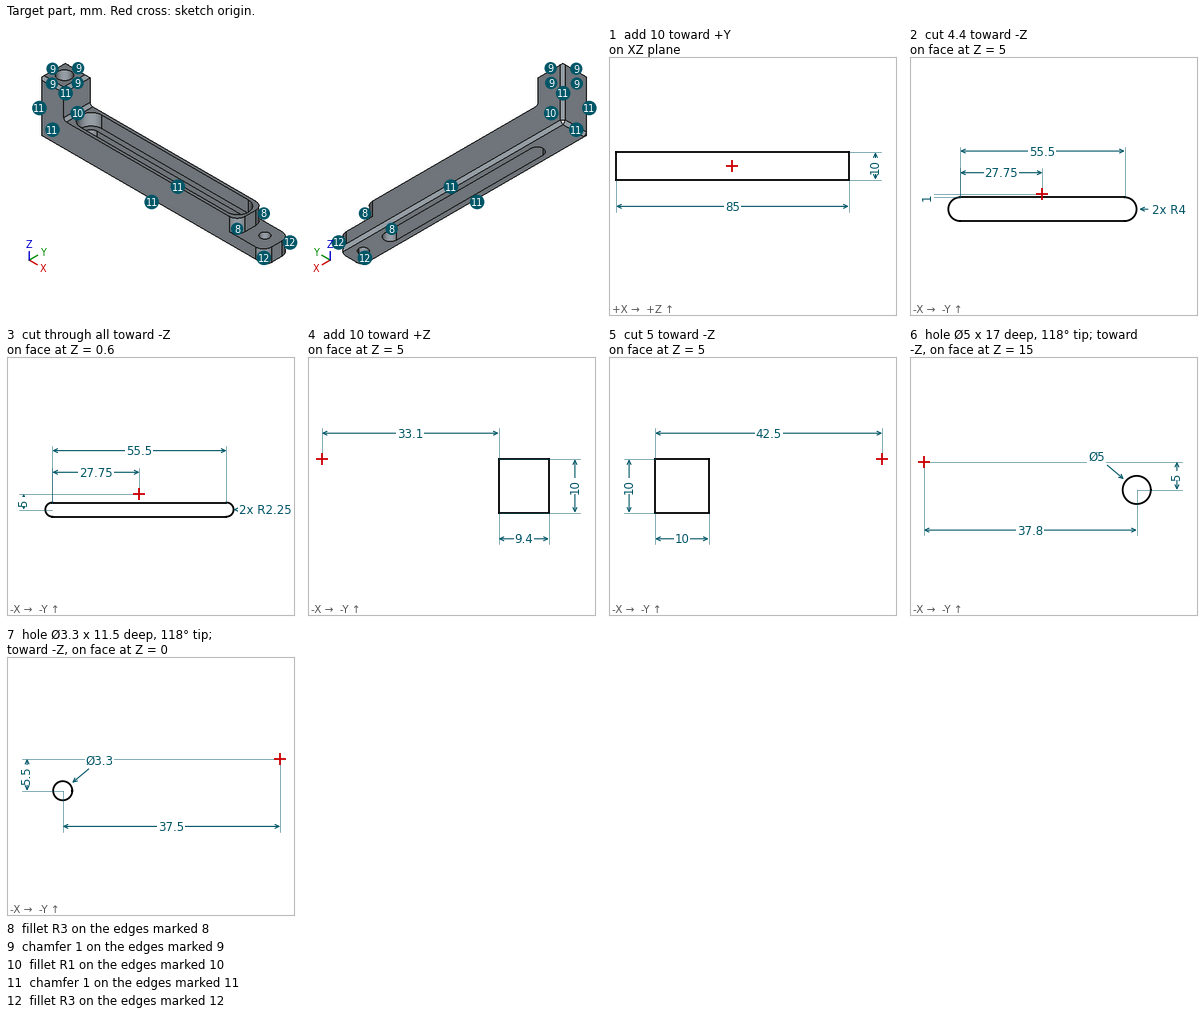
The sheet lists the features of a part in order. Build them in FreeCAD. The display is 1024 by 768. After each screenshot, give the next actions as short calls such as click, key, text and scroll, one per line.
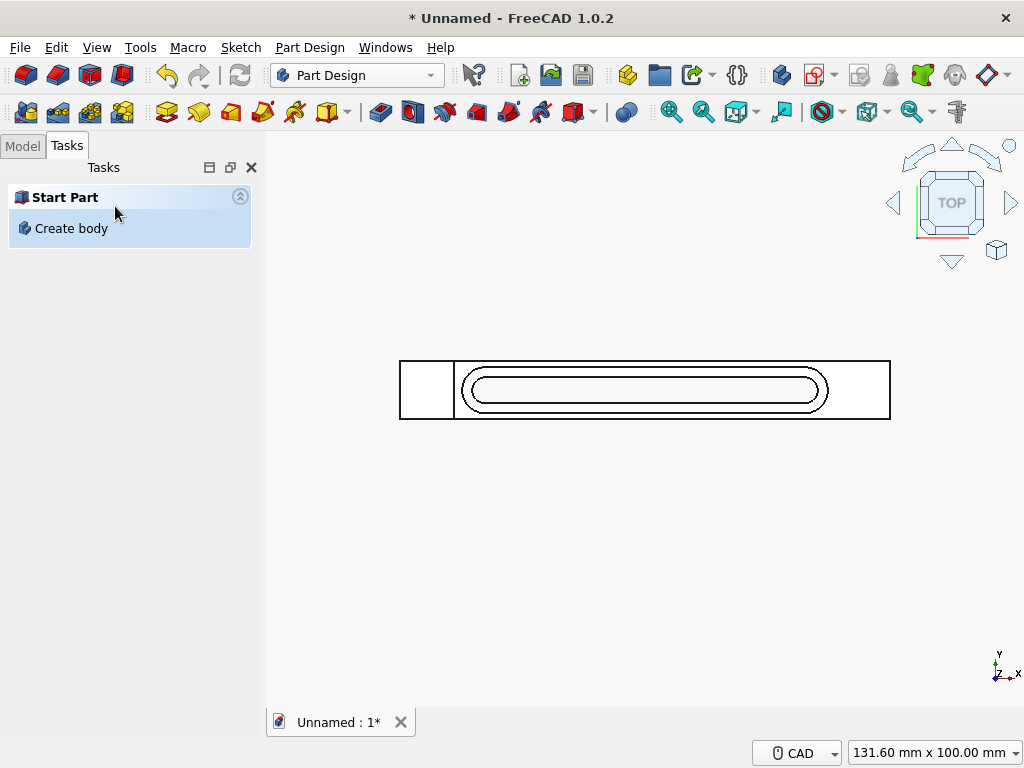
click(859, 389)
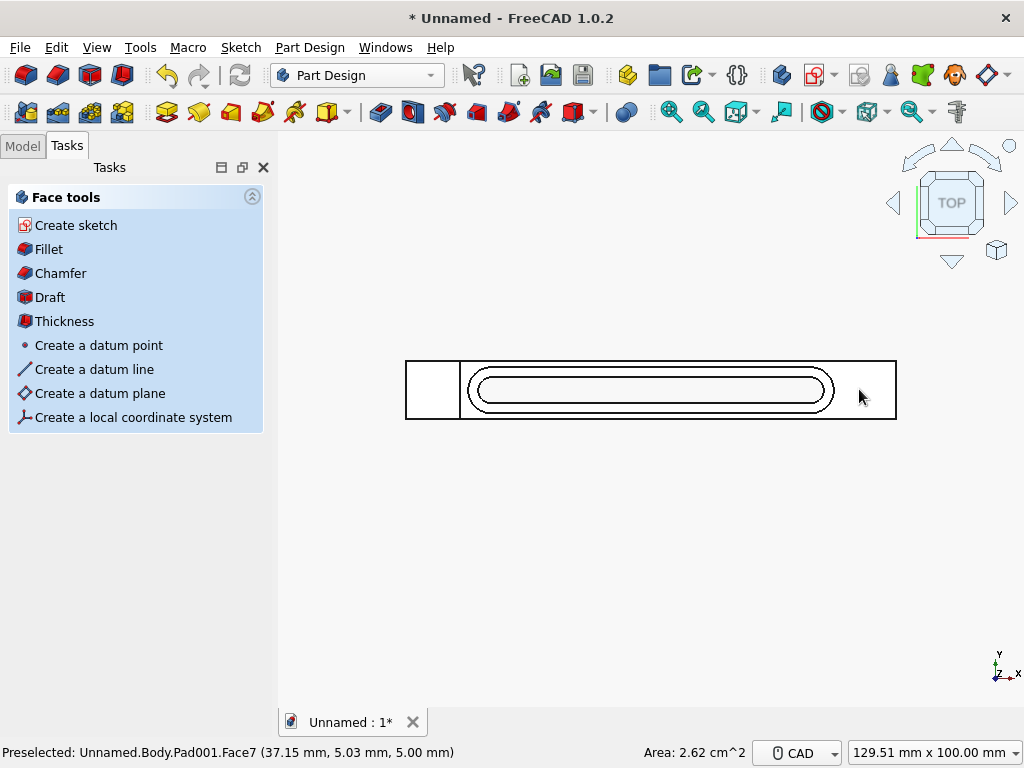
click(814, 76)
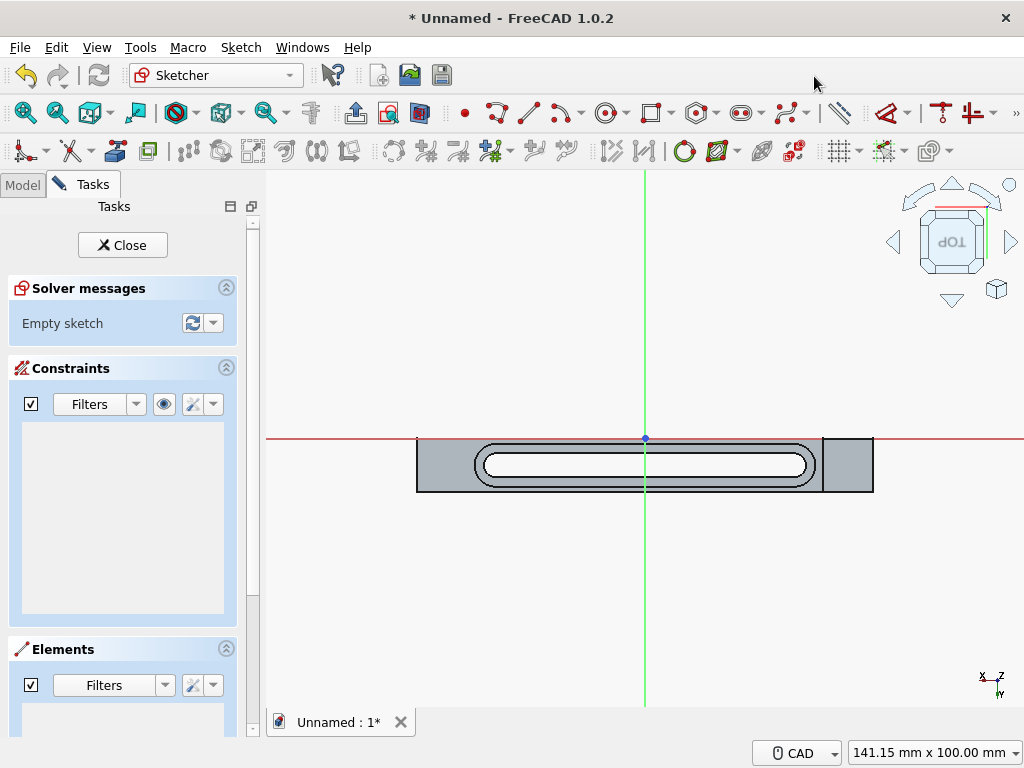
click(420, 114)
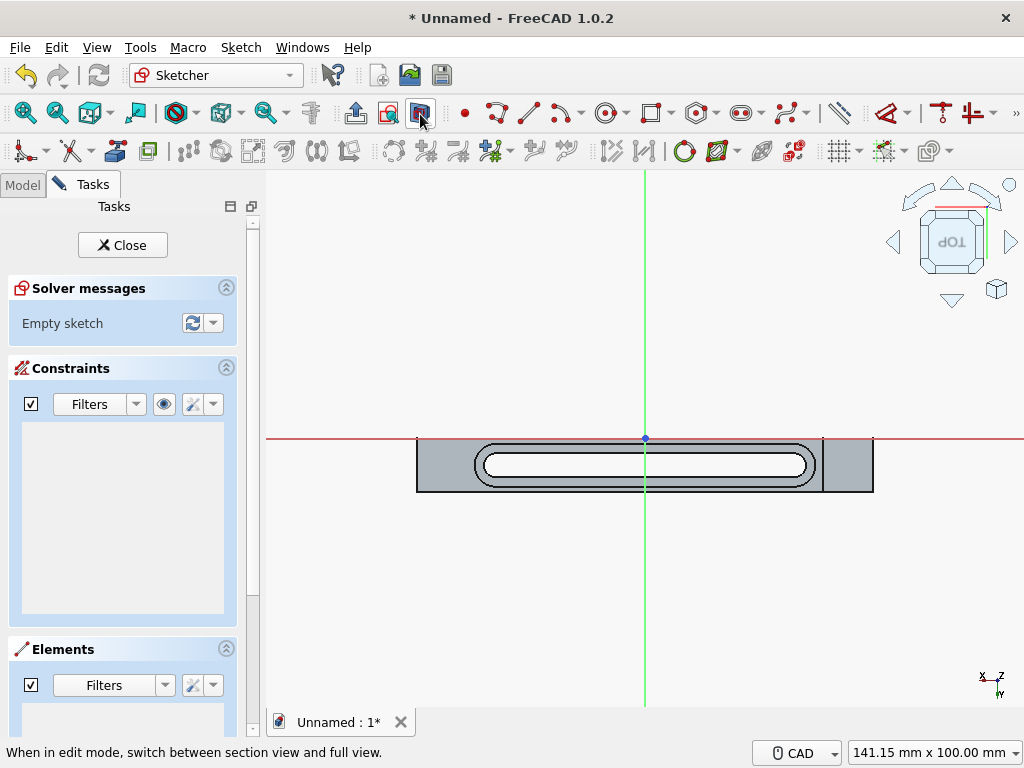
scroll(417, 471, up, 9)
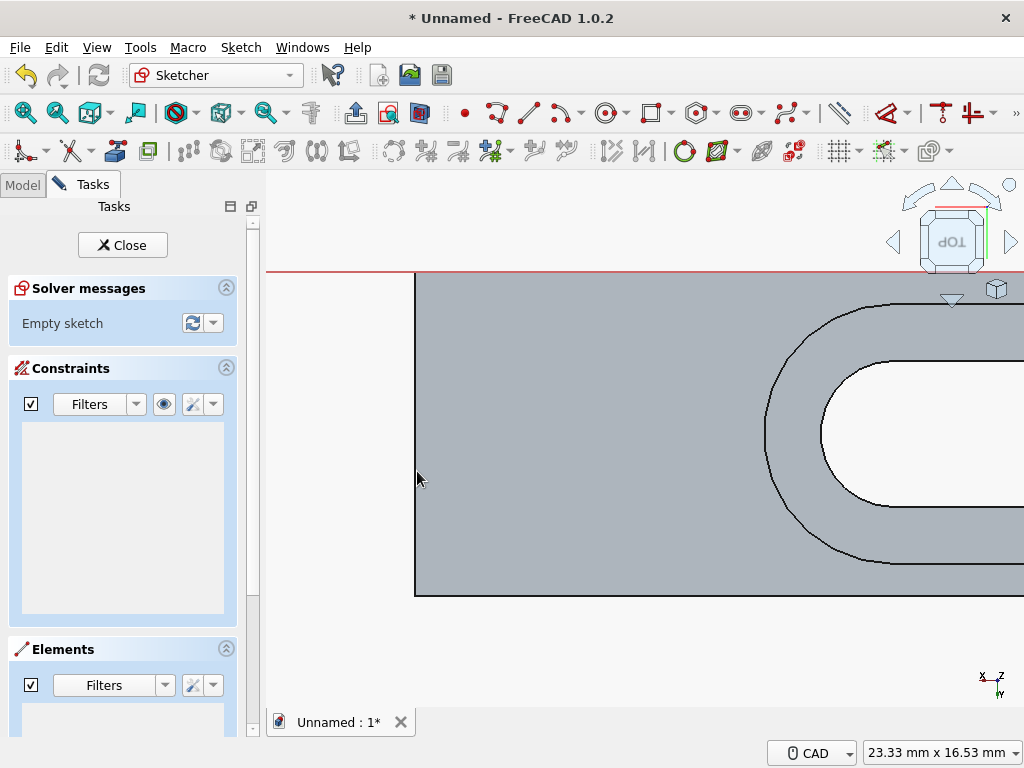
key(g)
key(r)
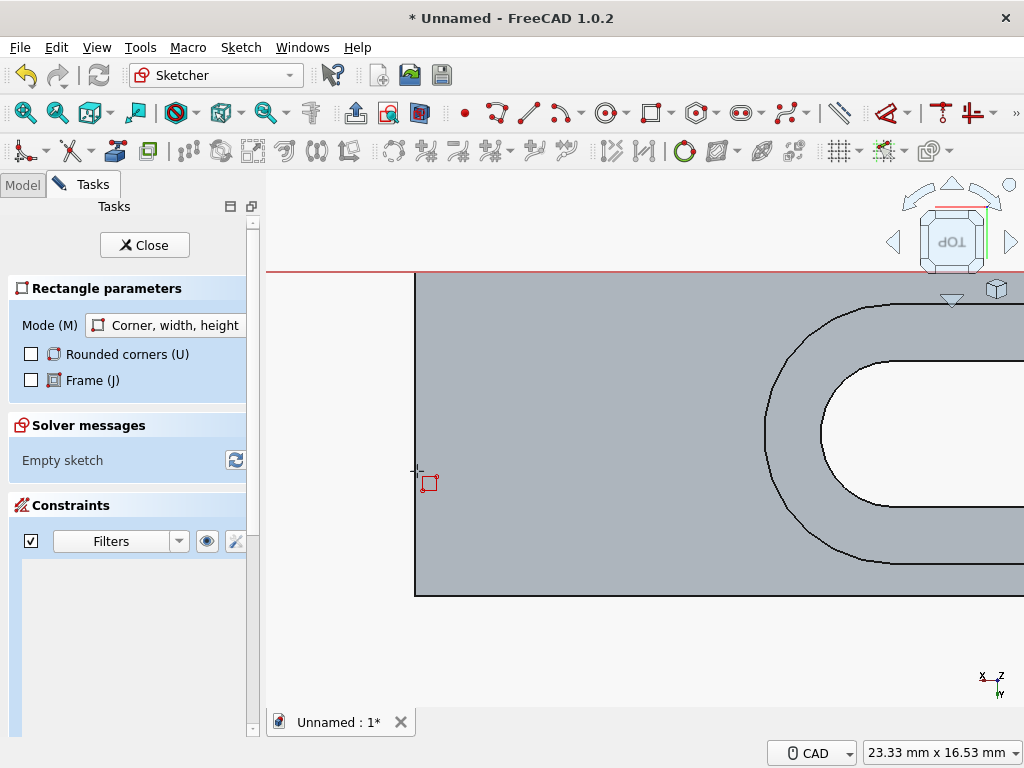
click(415, 272)
click(739, 596)
key(Escape)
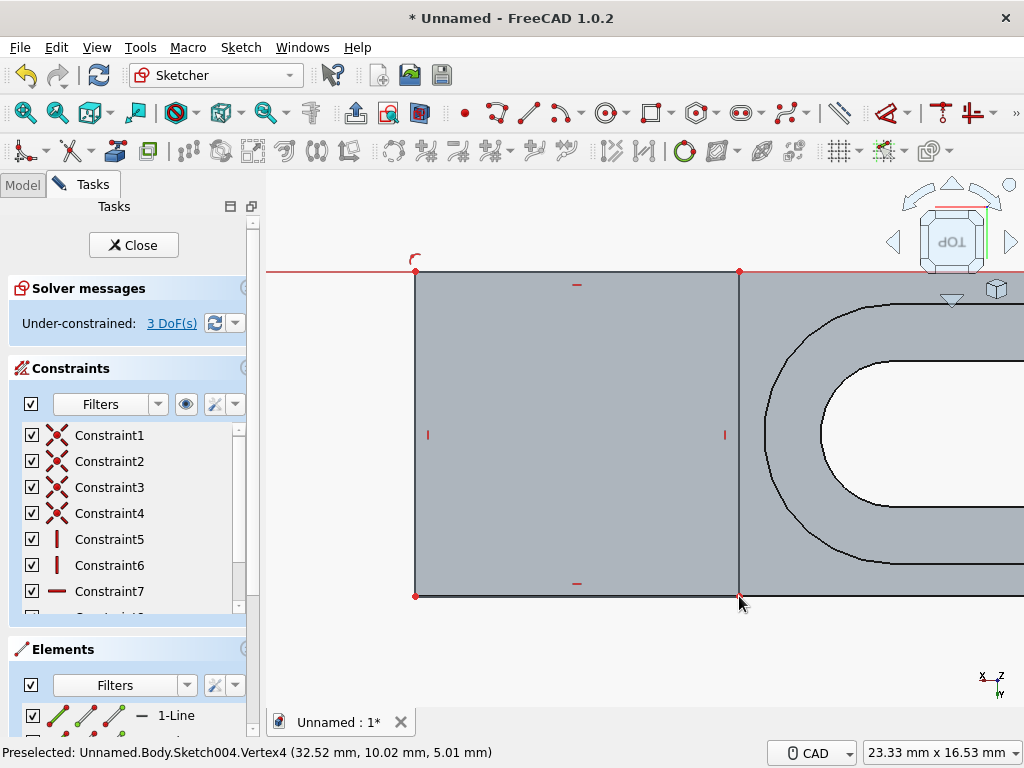
key(d)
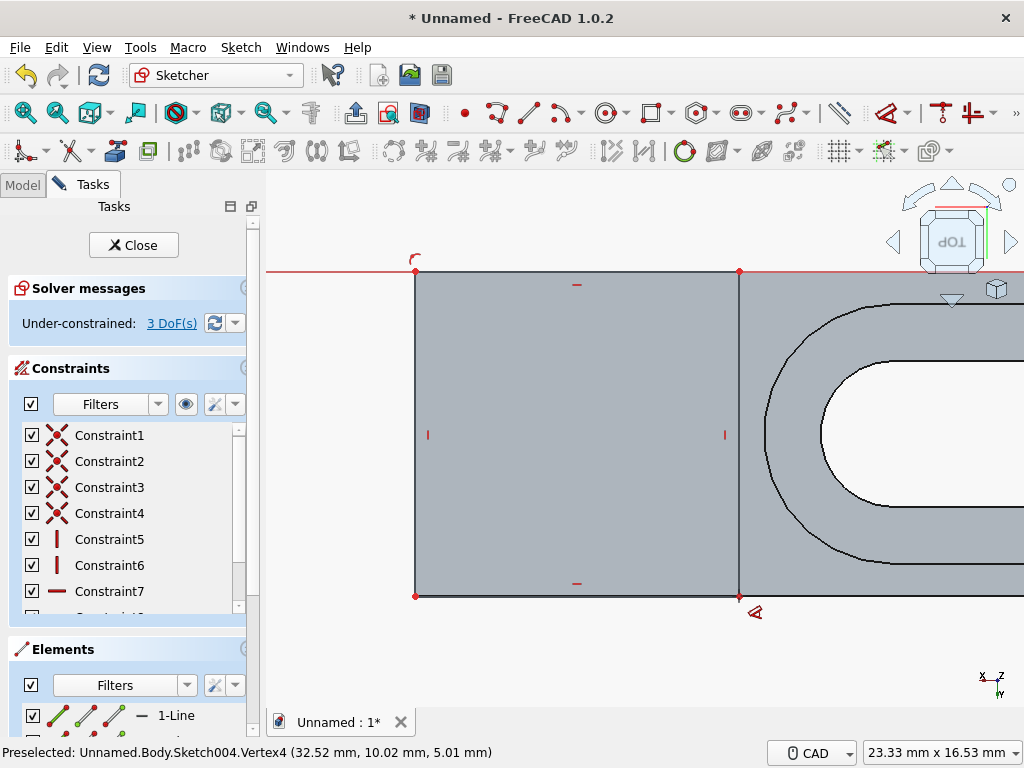
click(415, 369)
click(381, 434)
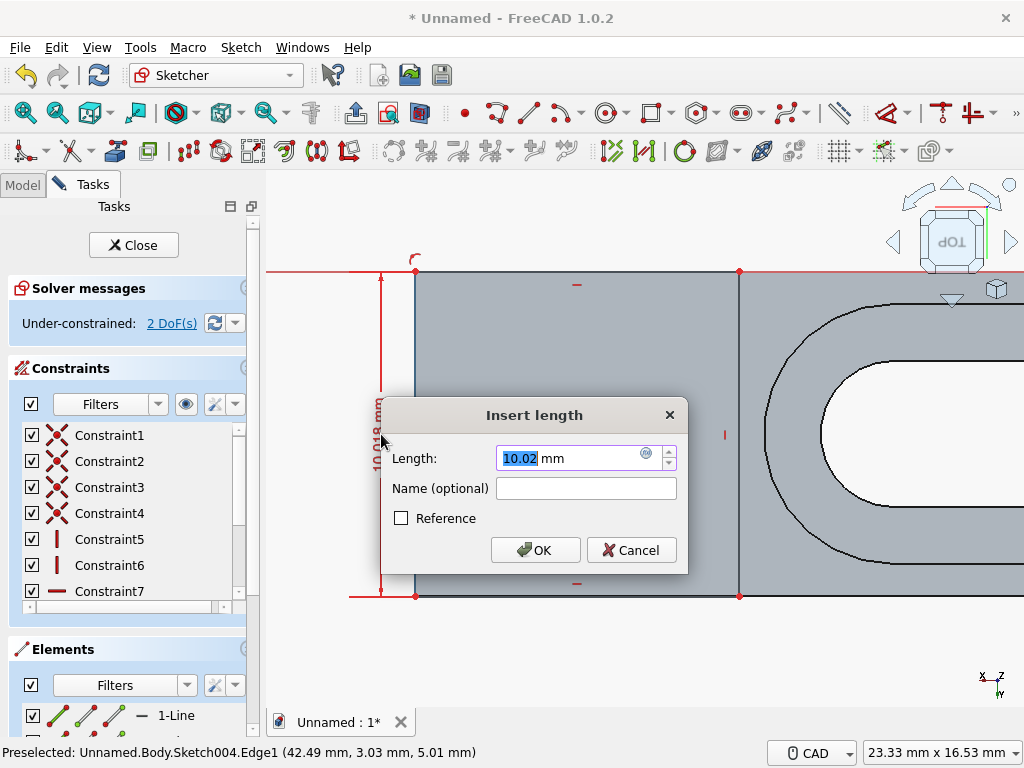
text(10)
key(Return)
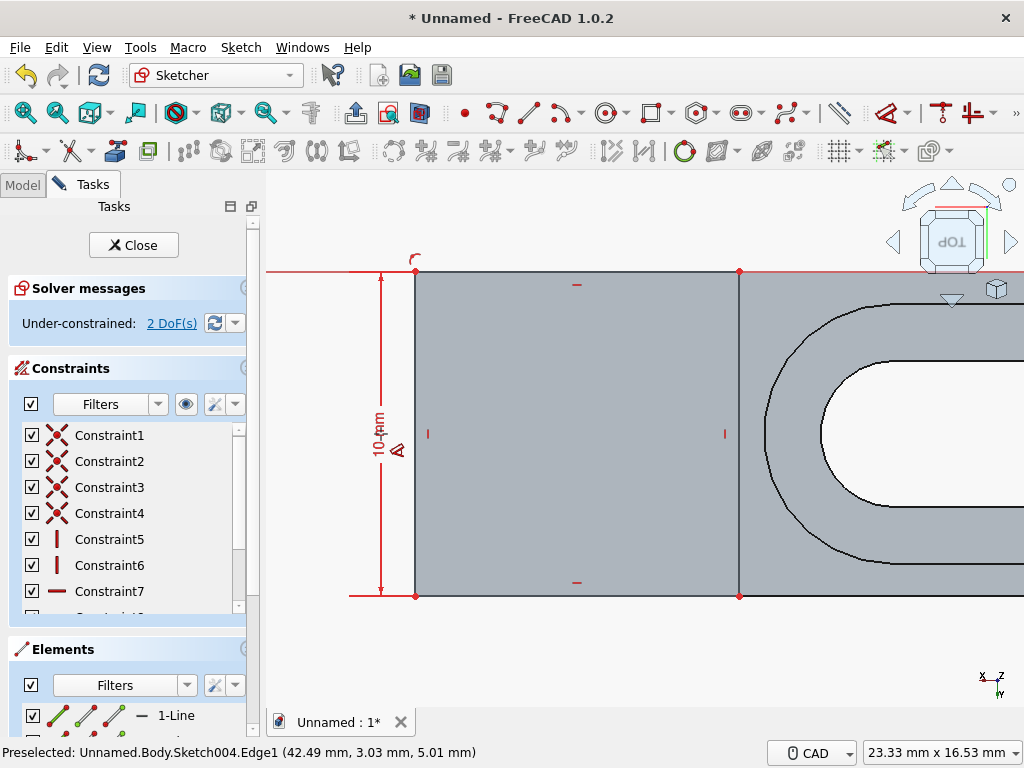
click(512, 596)
click(577, 630)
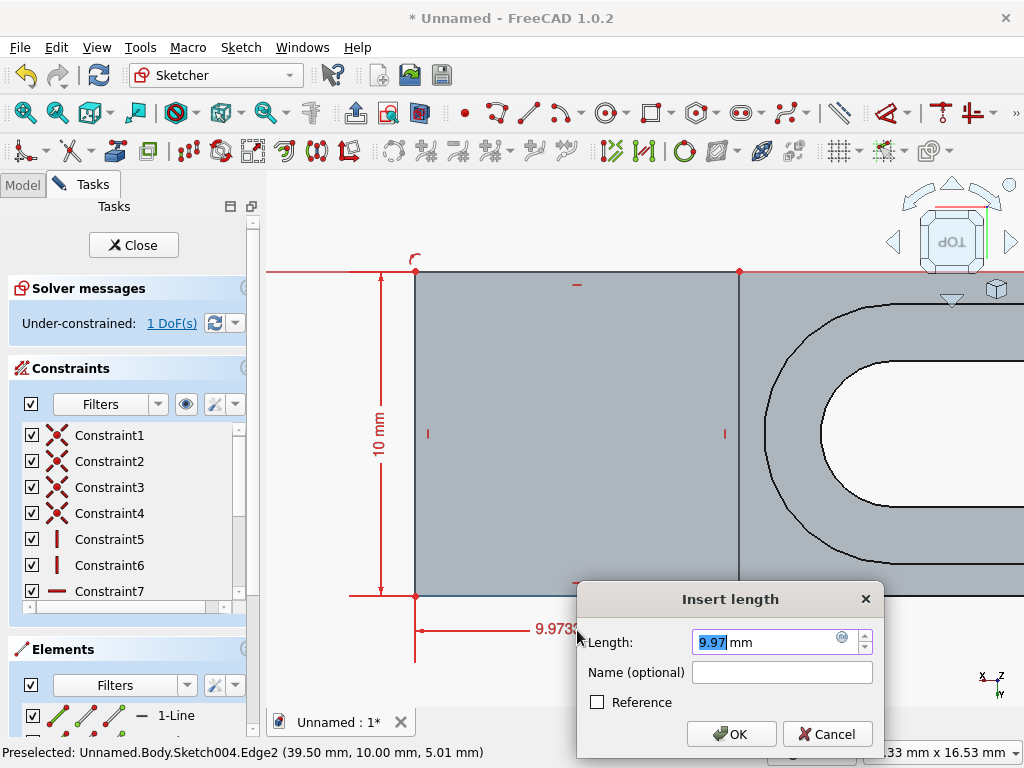
text(10)
key(Return)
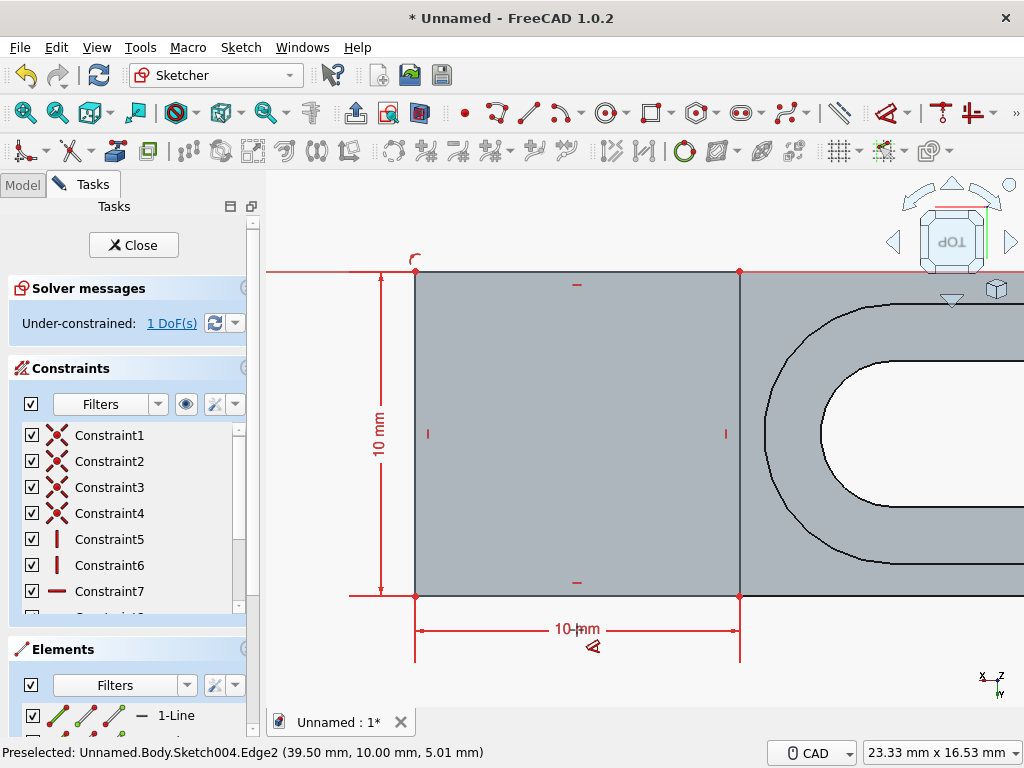
click(415, 272)
click(637, 238)